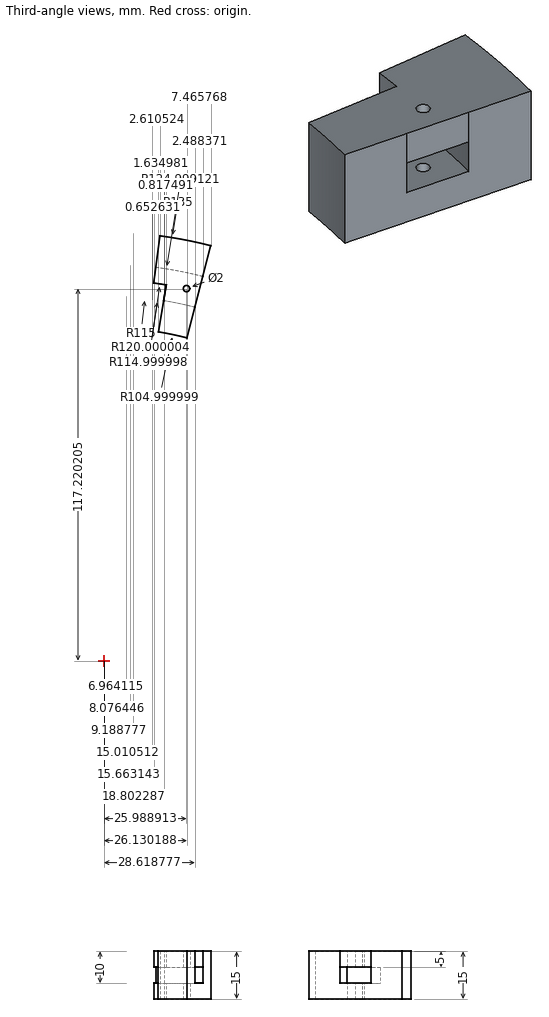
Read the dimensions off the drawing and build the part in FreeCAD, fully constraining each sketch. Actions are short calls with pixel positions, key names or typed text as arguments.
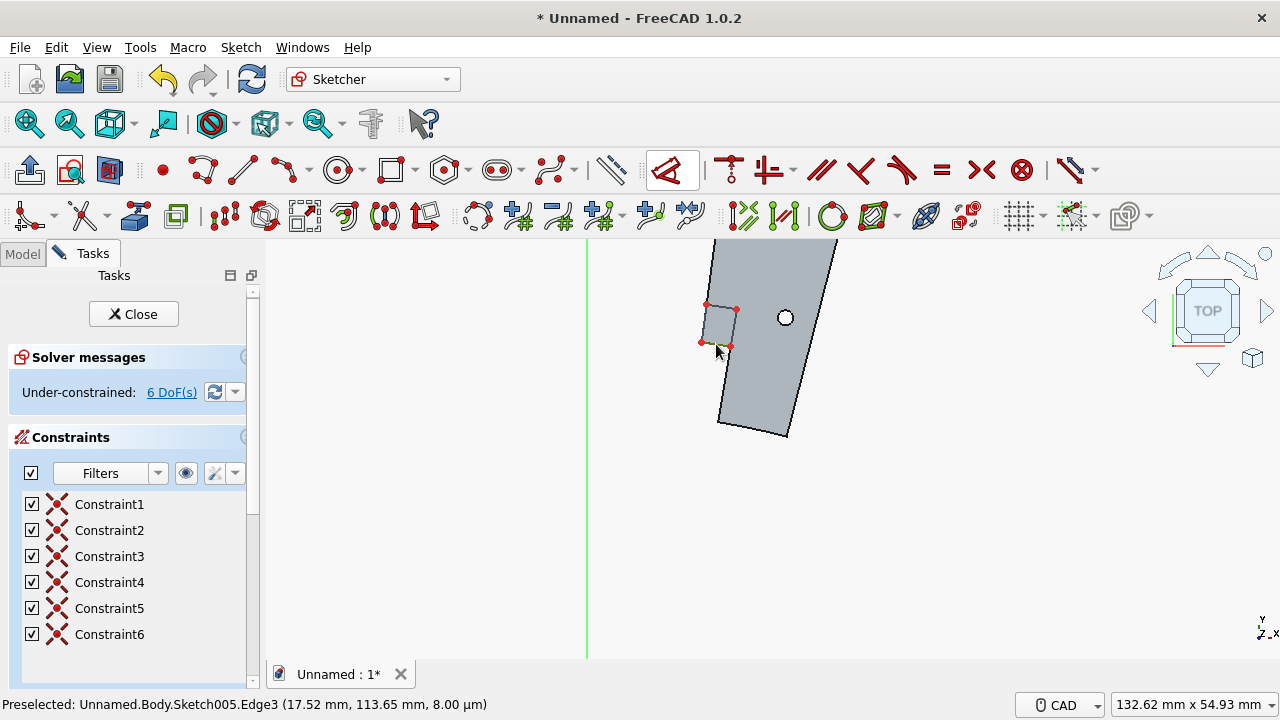
click(694, 170)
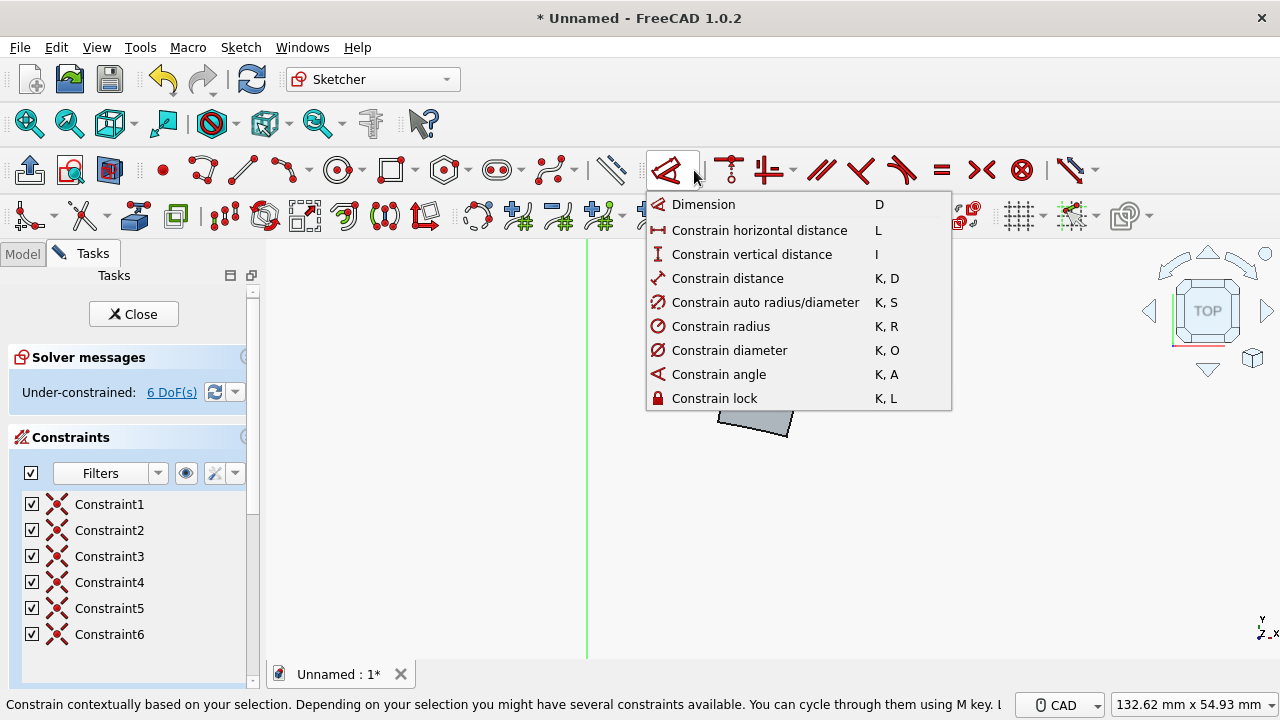
click(799, 326)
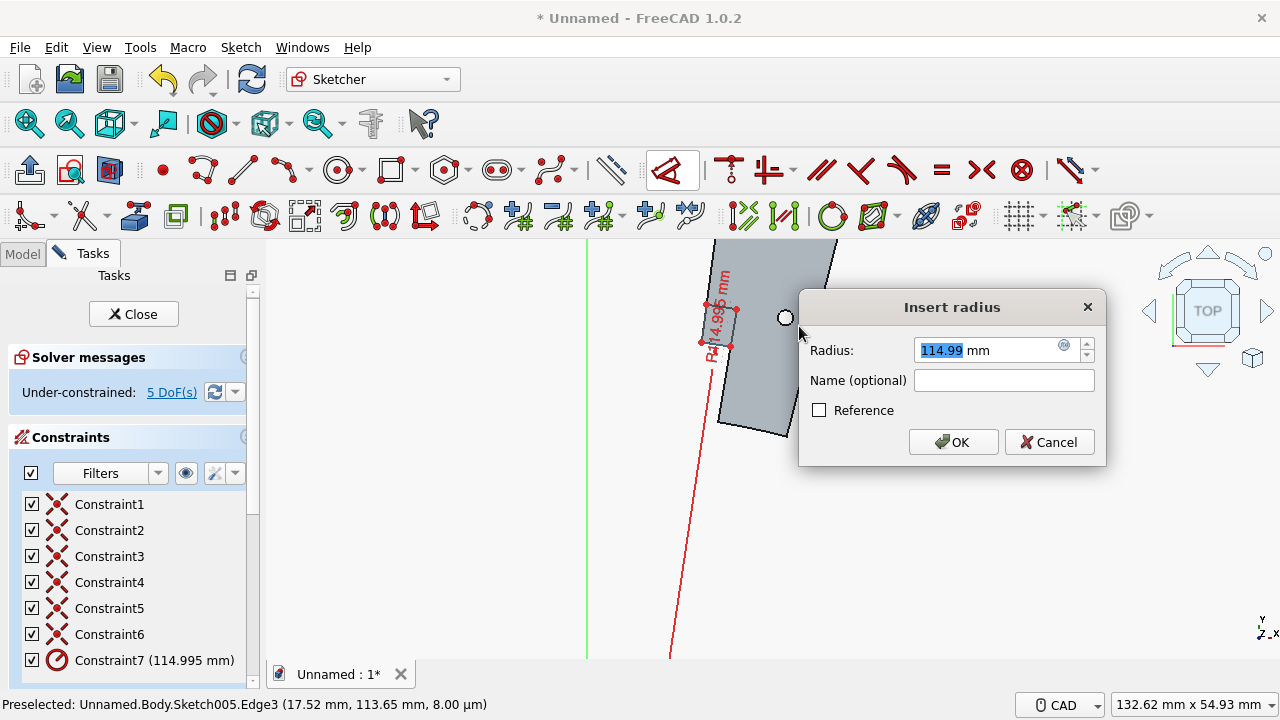
text(114.999998)
key(Return)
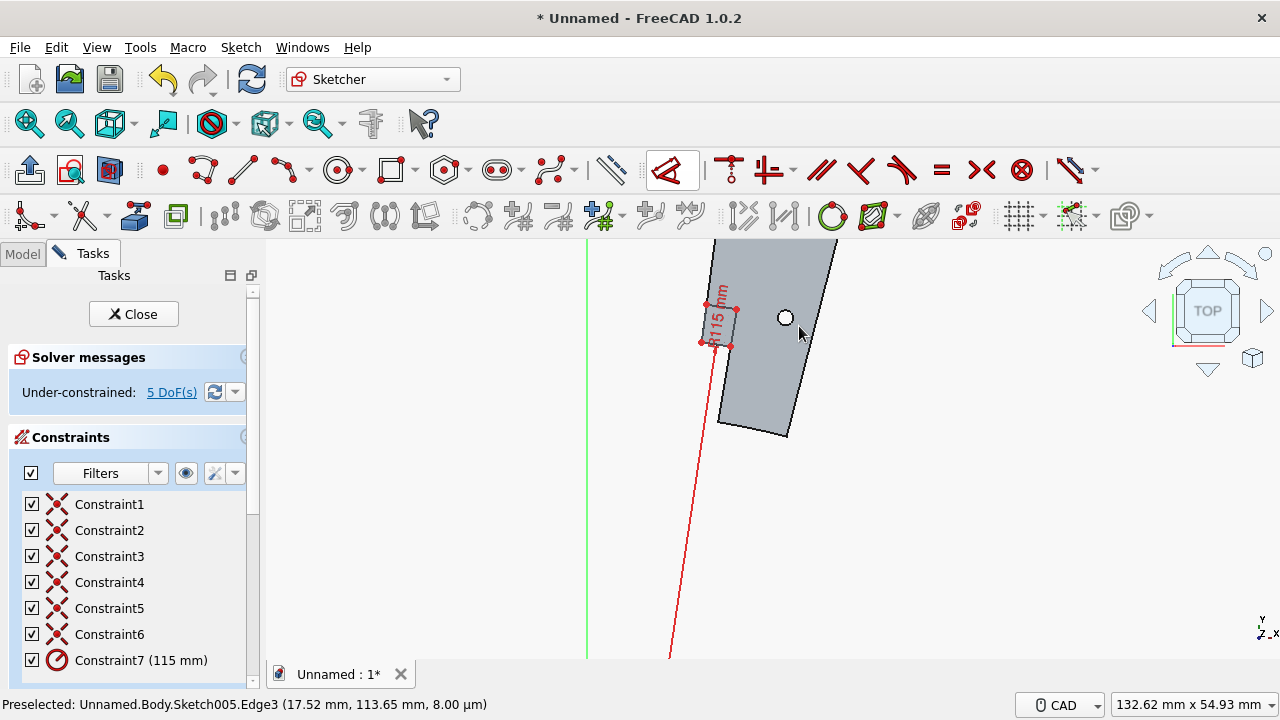
scroll(728, 308, up, 3)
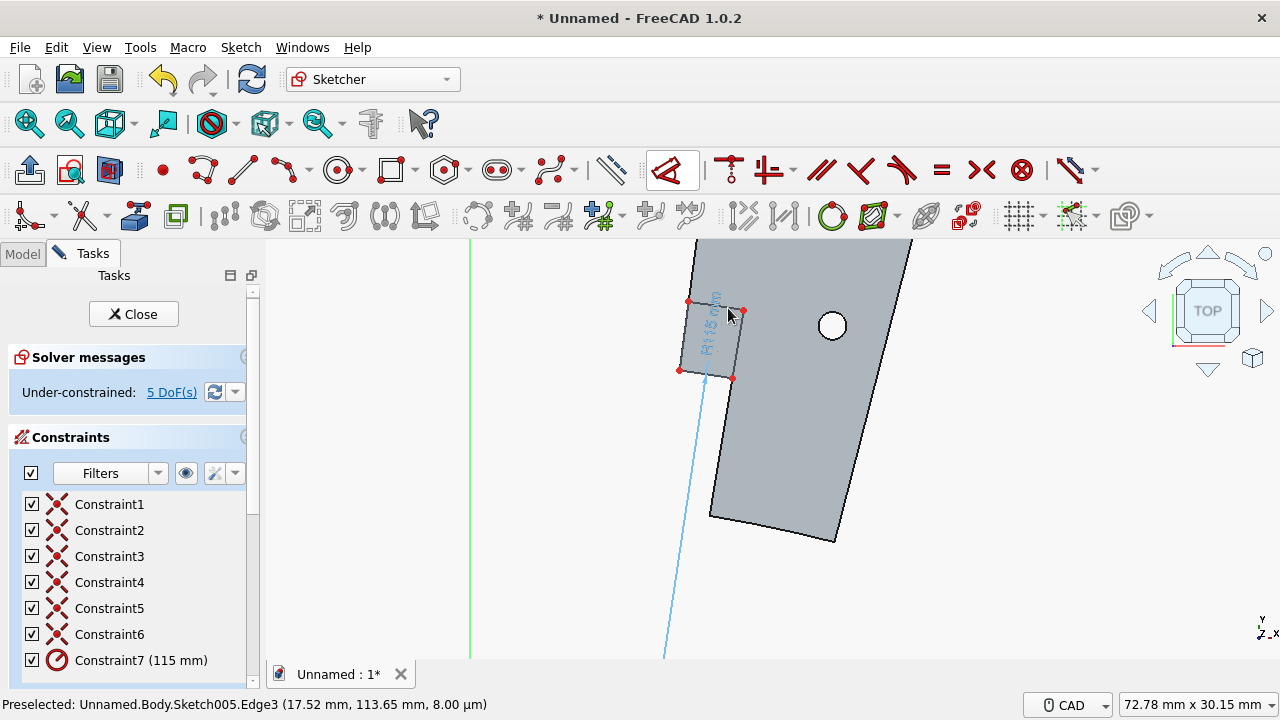
click(727, 307)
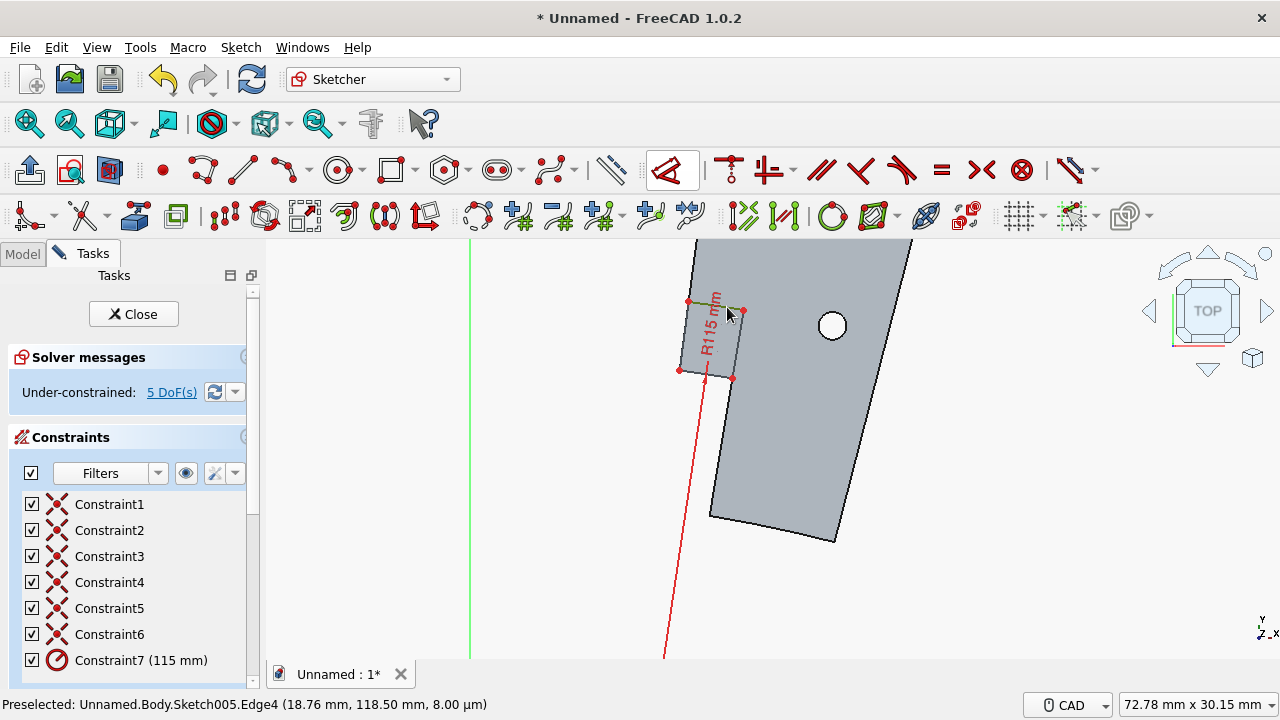
click(694, 170)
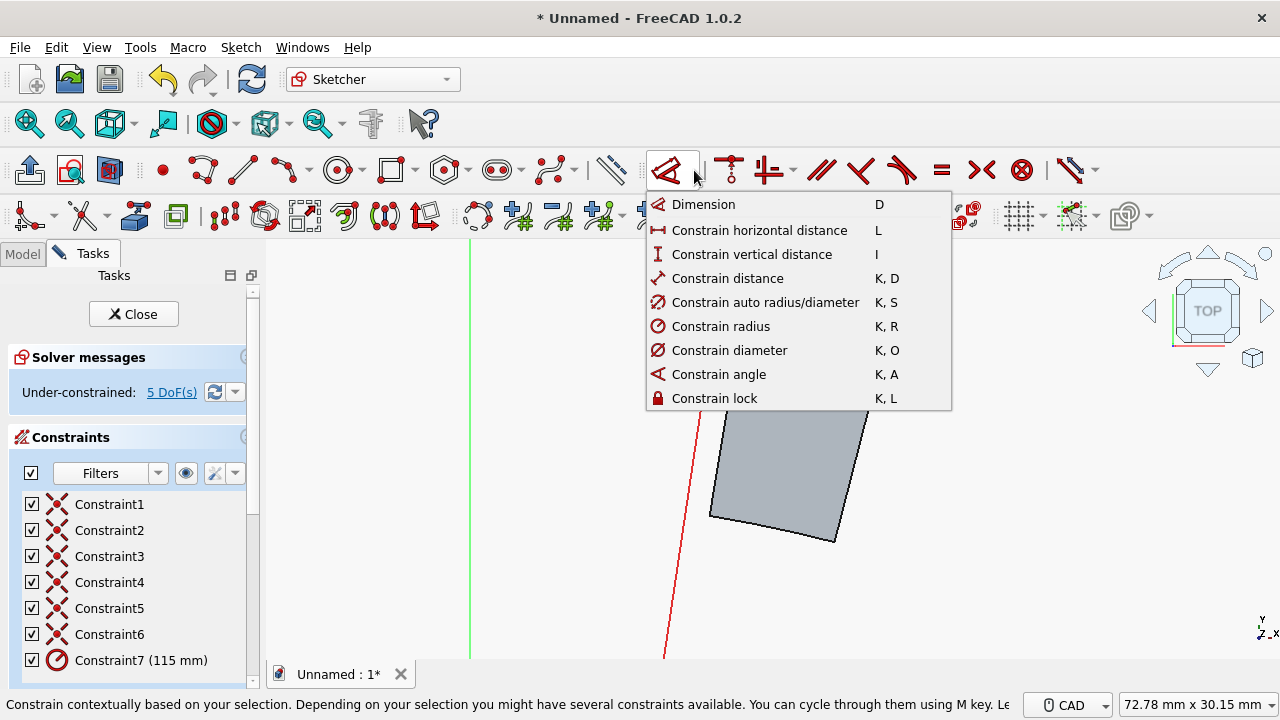
click(799, 326)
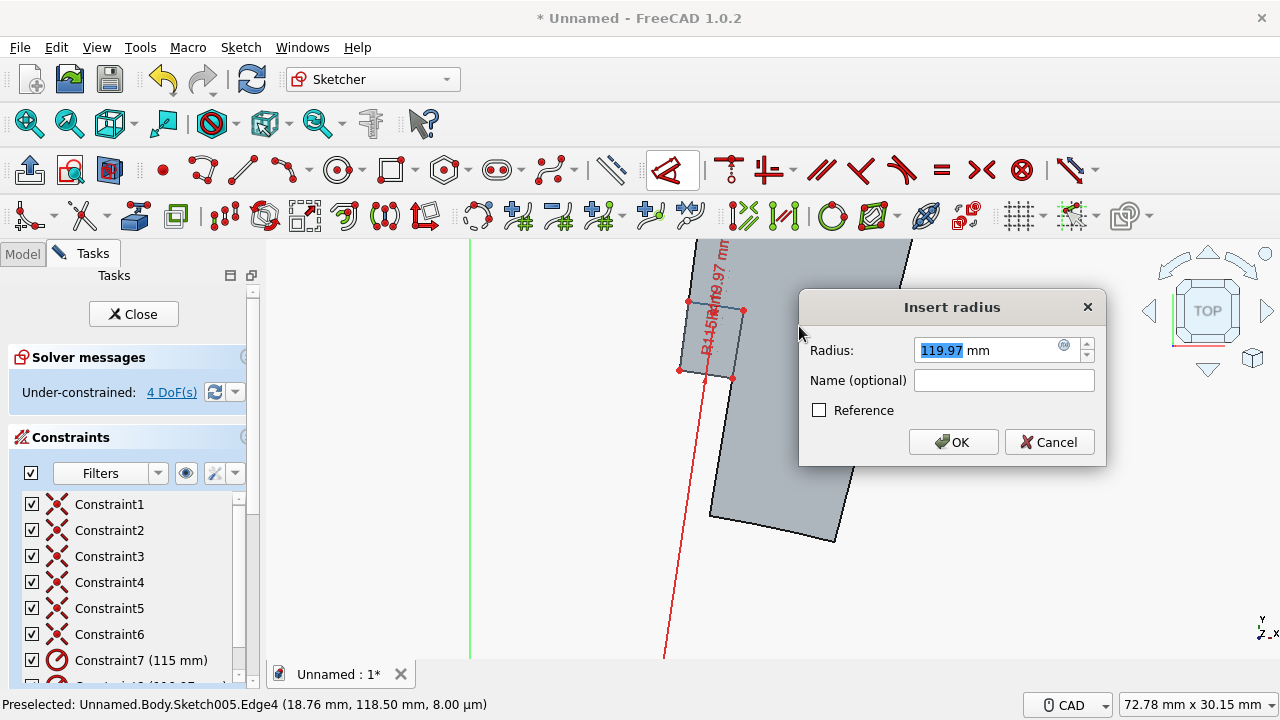
text(120.000004)
key(Return)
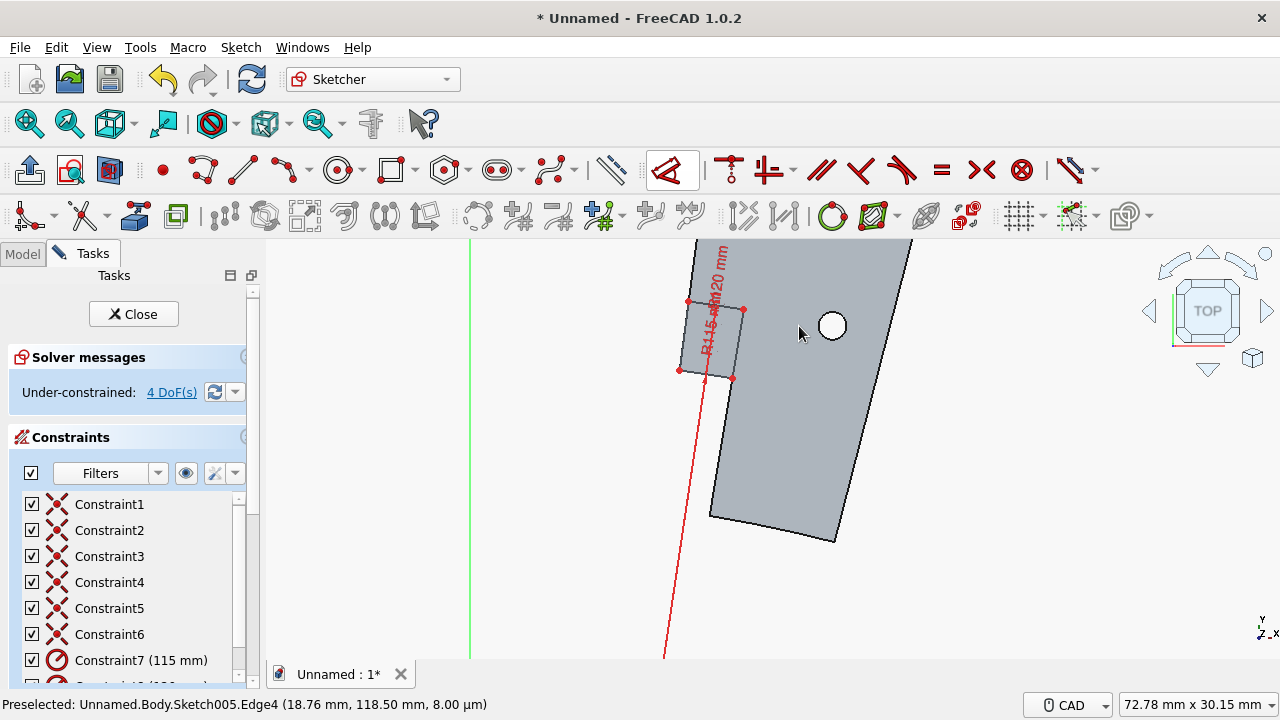
scroll(686, 322, up, 8)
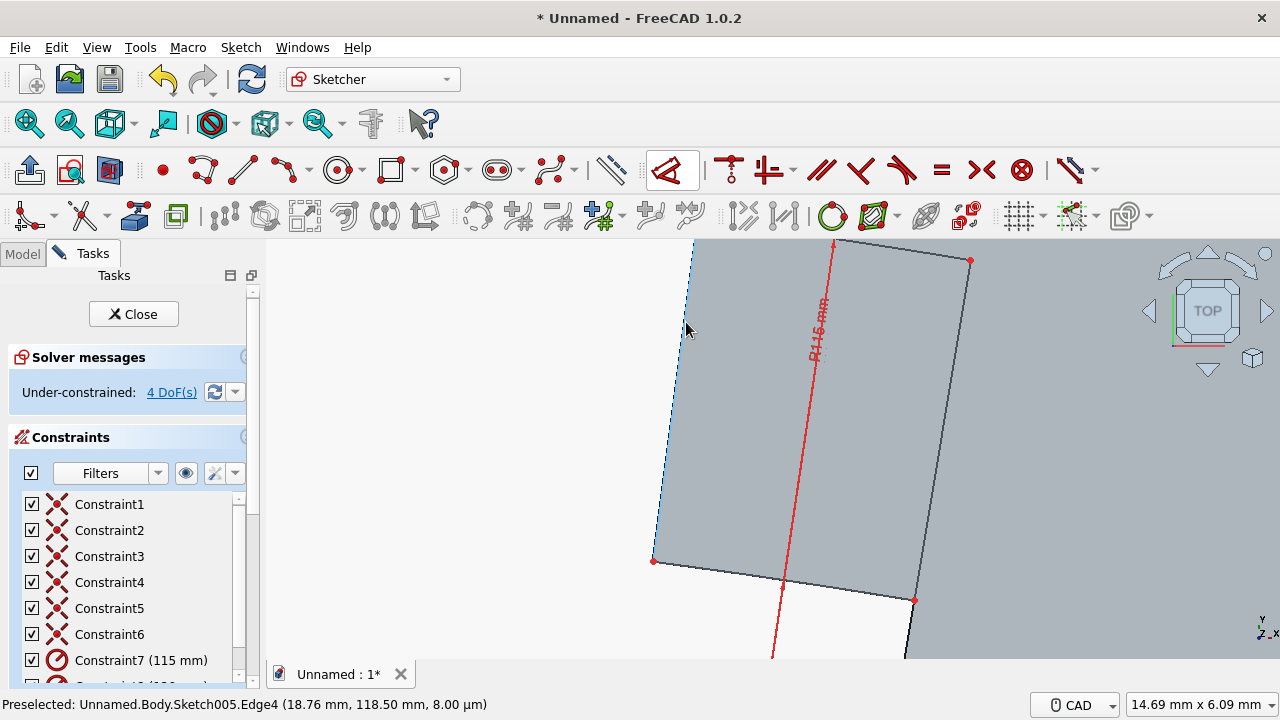
click(685, 322)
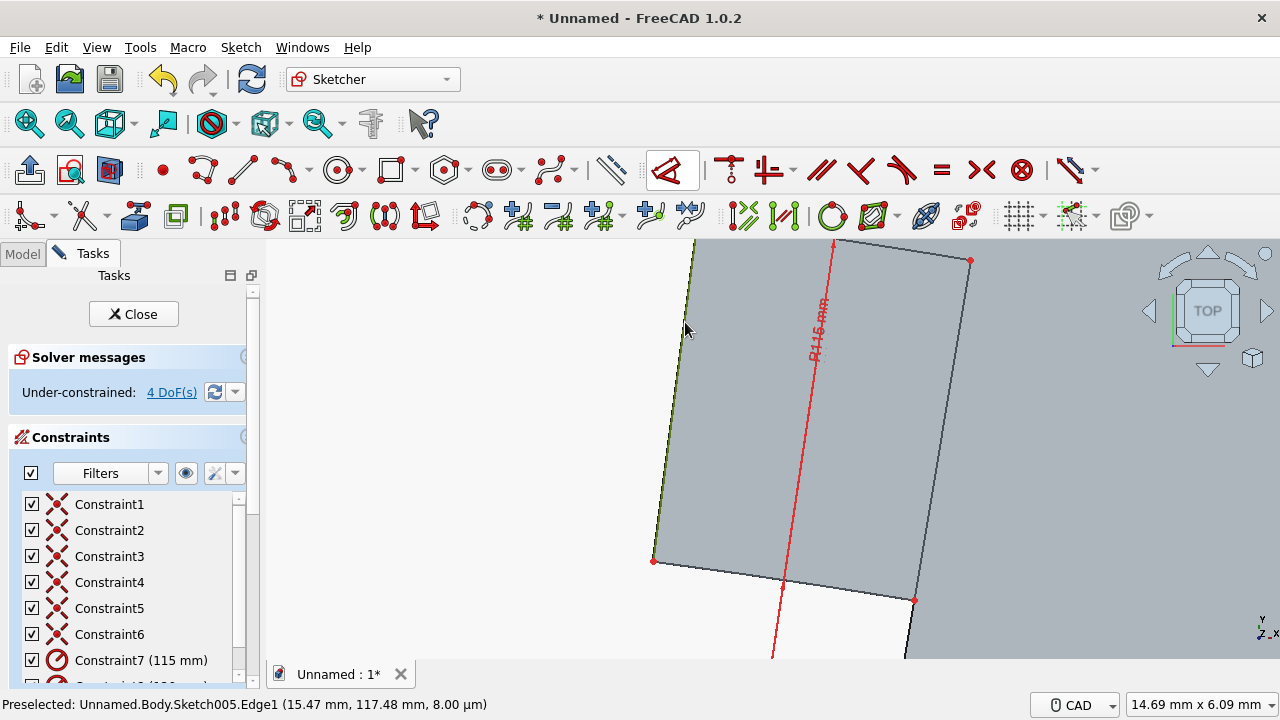
click(694, 170)